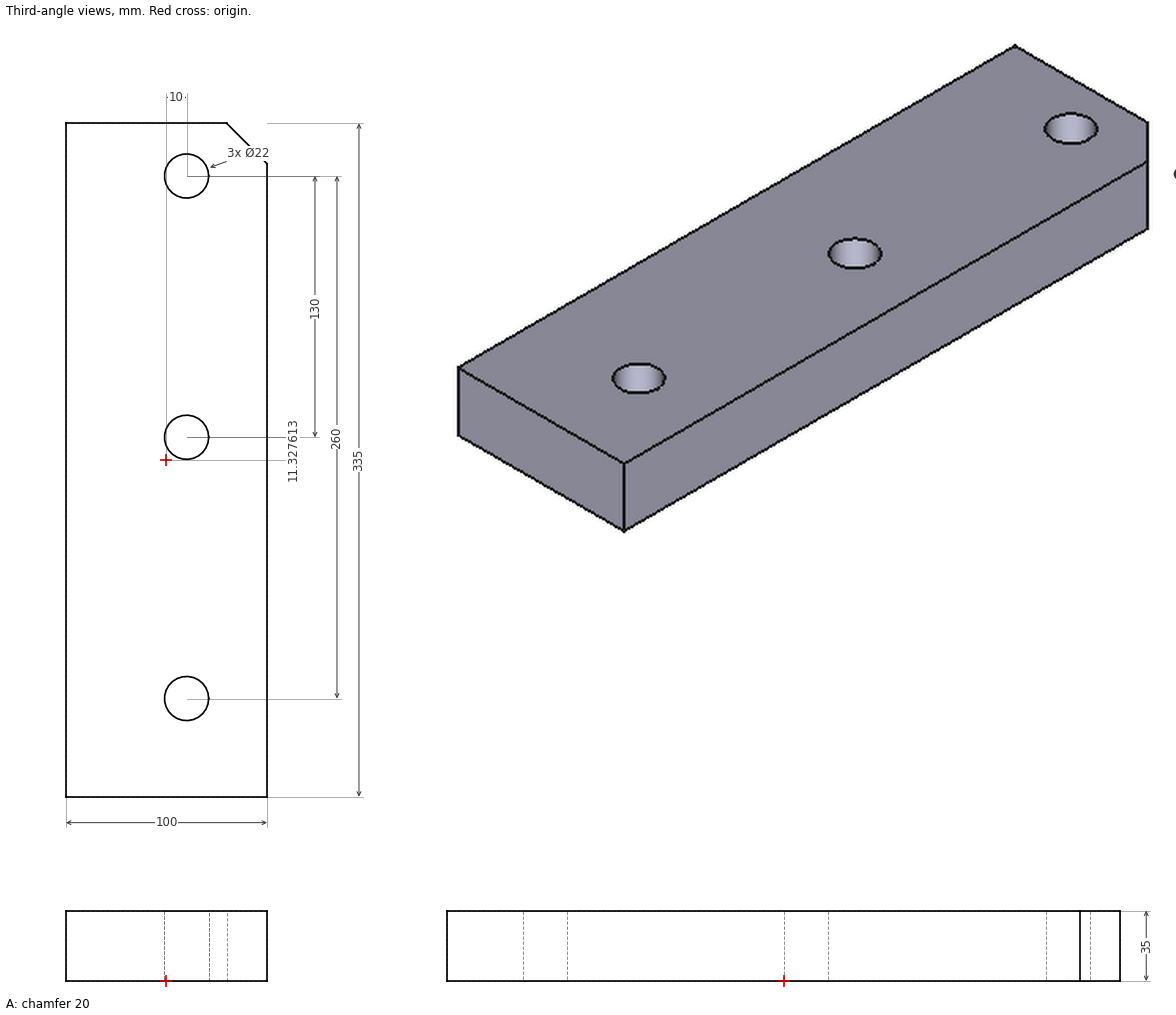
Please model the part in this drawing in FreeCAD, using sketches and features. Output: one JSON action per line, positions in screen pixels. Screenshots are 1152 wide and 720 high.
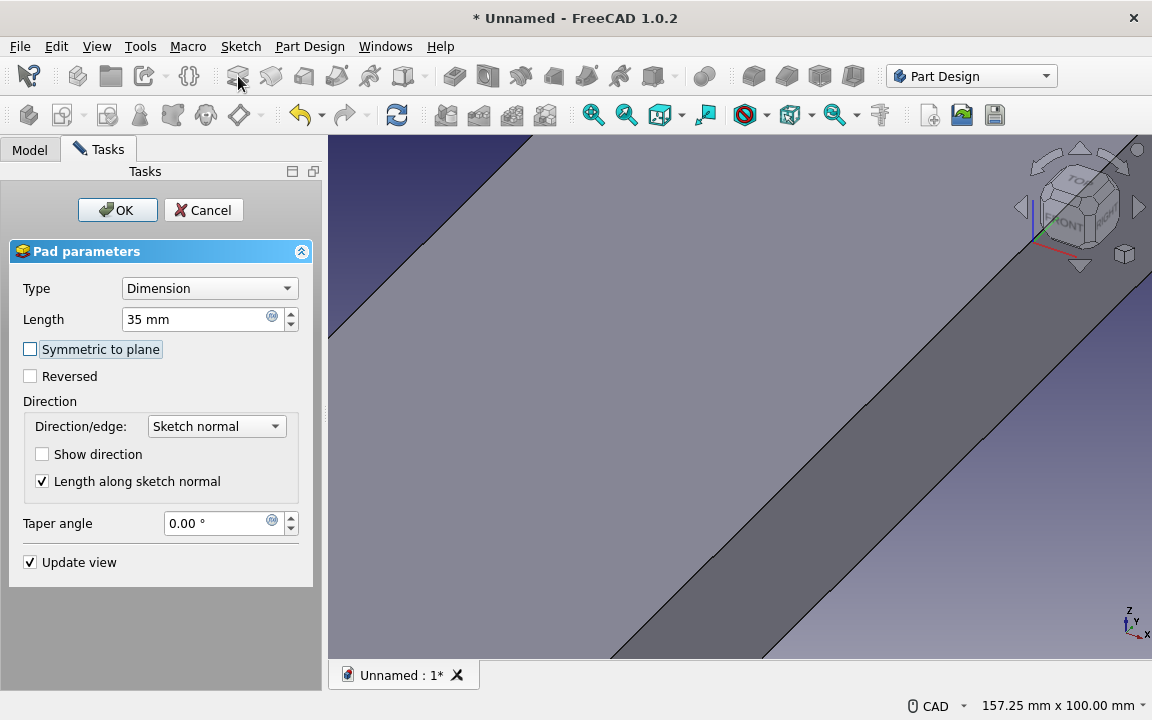
{"action": "left_click", "coordinate": [118, 210]}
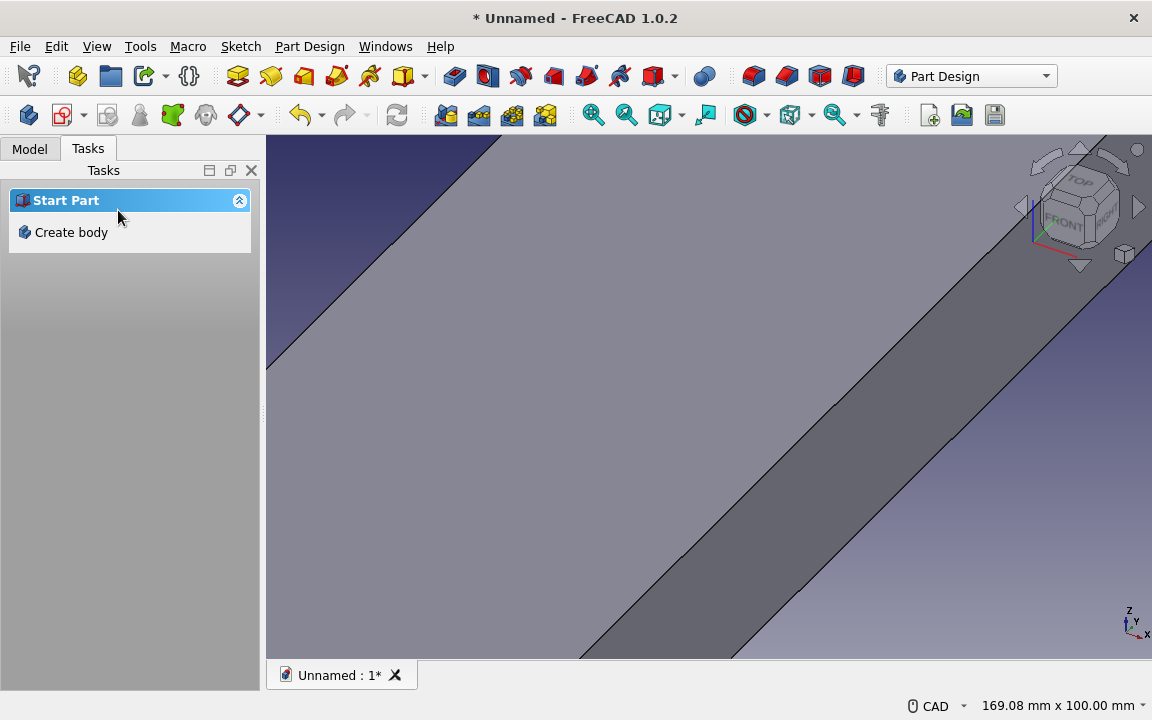
{"action": "left_click", "coordinate": [594, 116]}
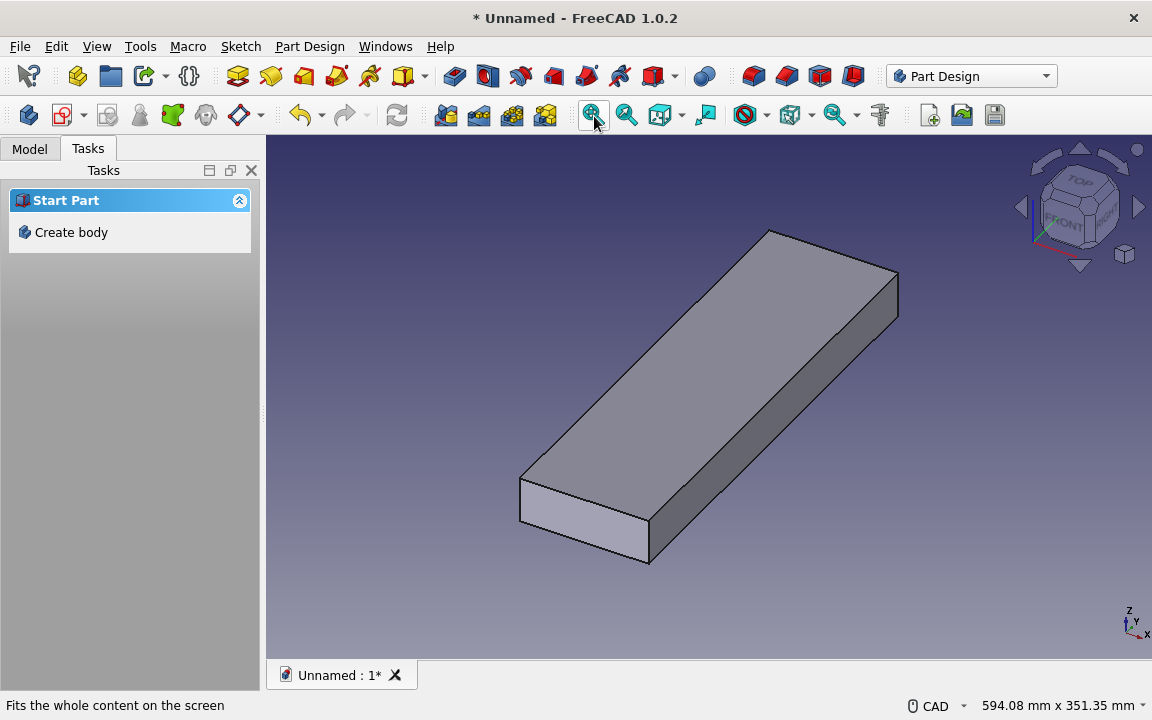
{"action": "key", "text": "0"}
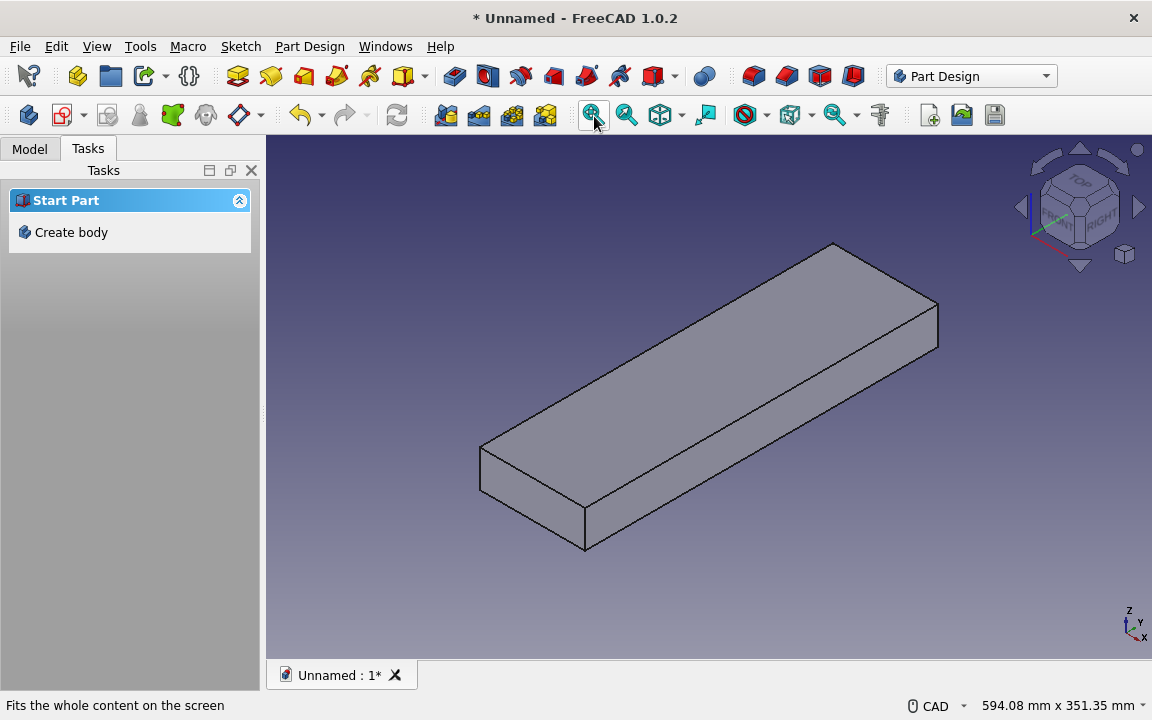
{"action": "key", "text": "2"}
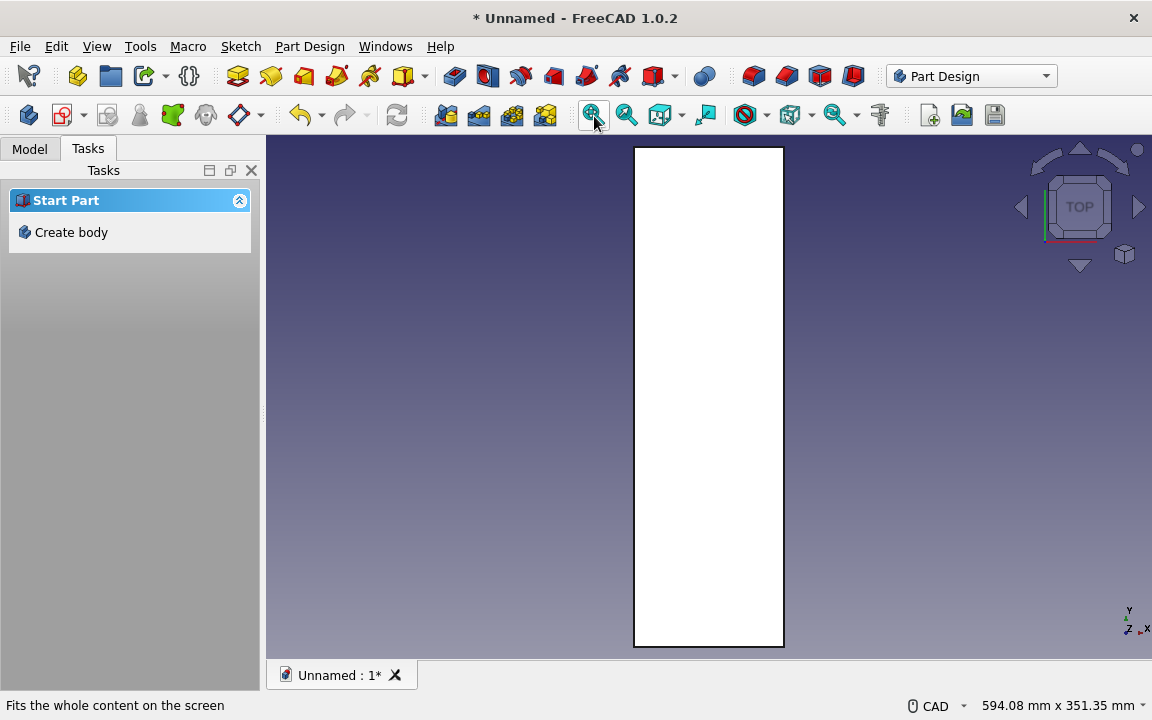
{"action": "key", "text": "1"}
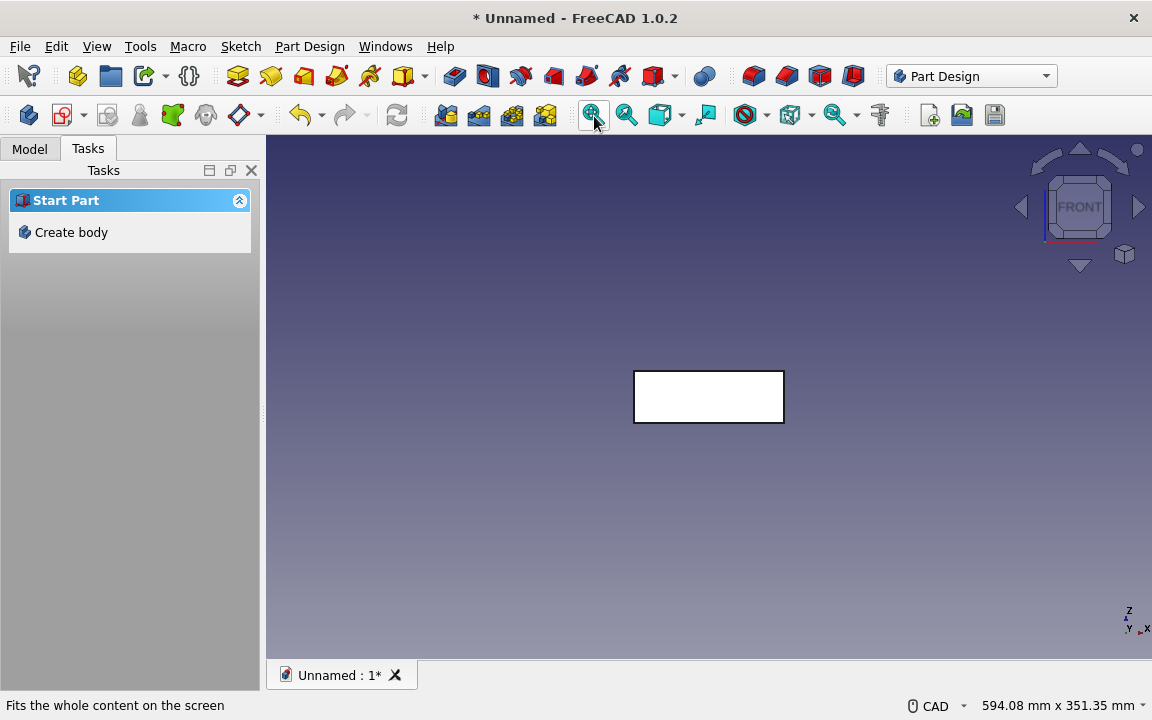
{"action": "left_click", "coordinate": [594, 116]}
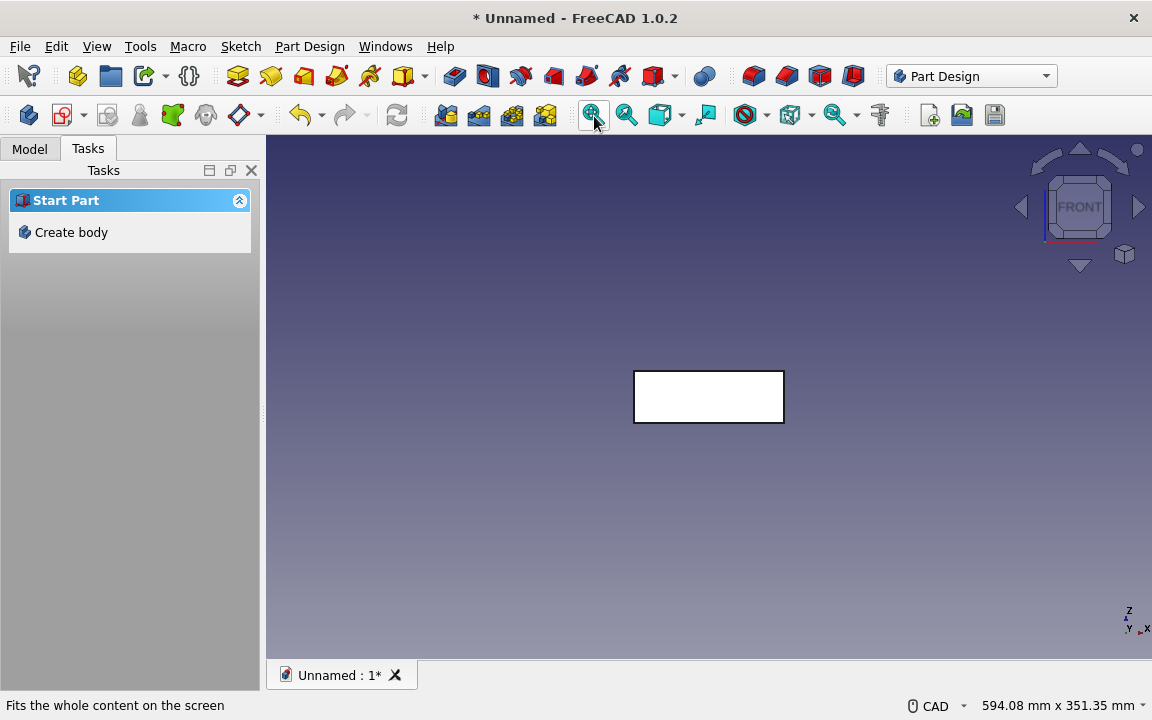
{"action": "key", "text": "3"}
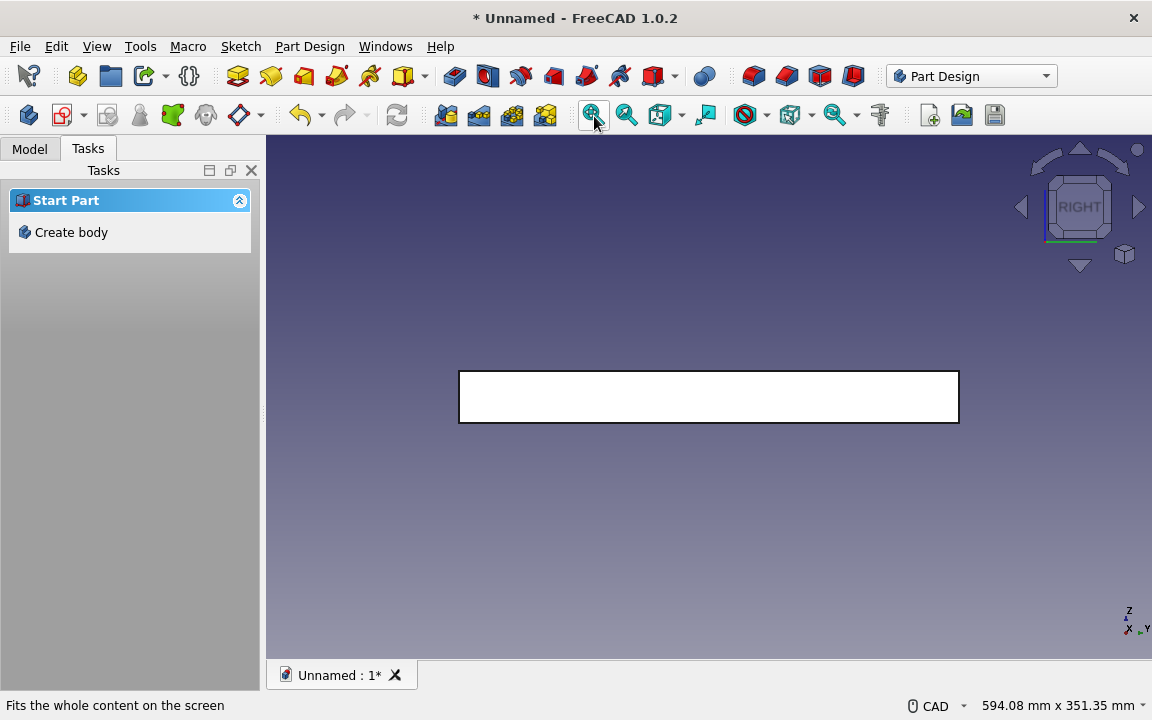
{"action": "left_click", "coordinate": [959, 396]}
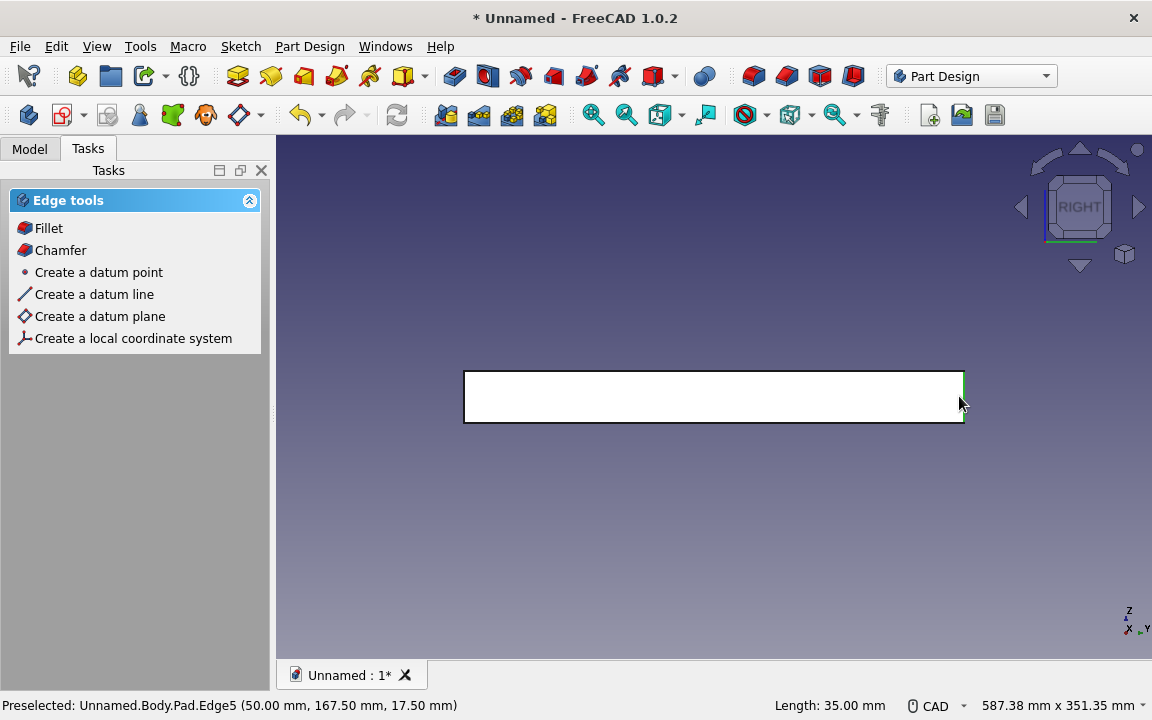
{"action": "left_click", "coordinate": [787, 76]}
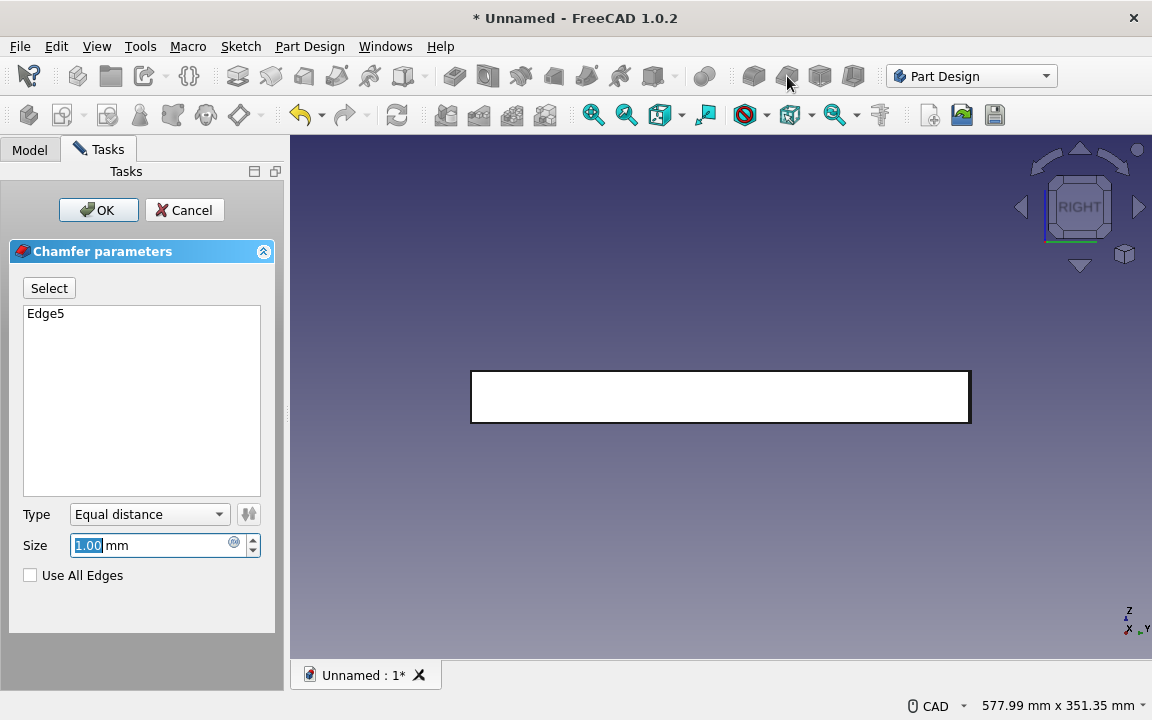
{"action": "type", "text": "20"}
{"action": "key", "text": "Tab"}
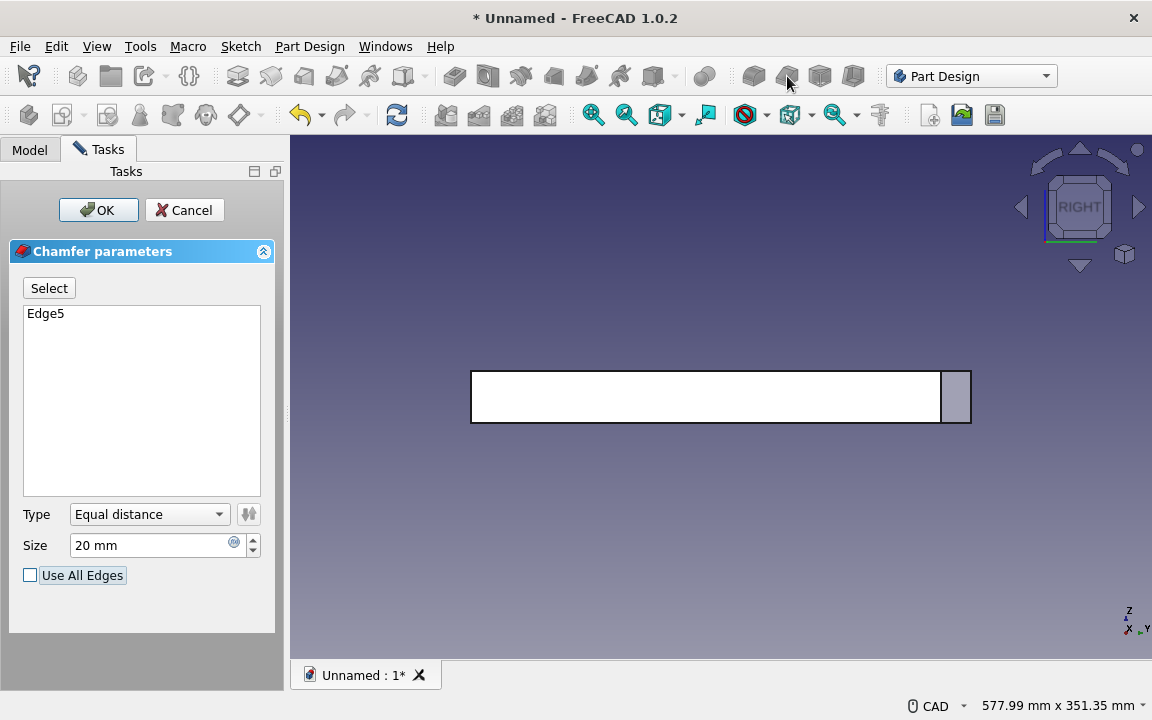
{"action": "left_click", "coordinate": [99, 210]}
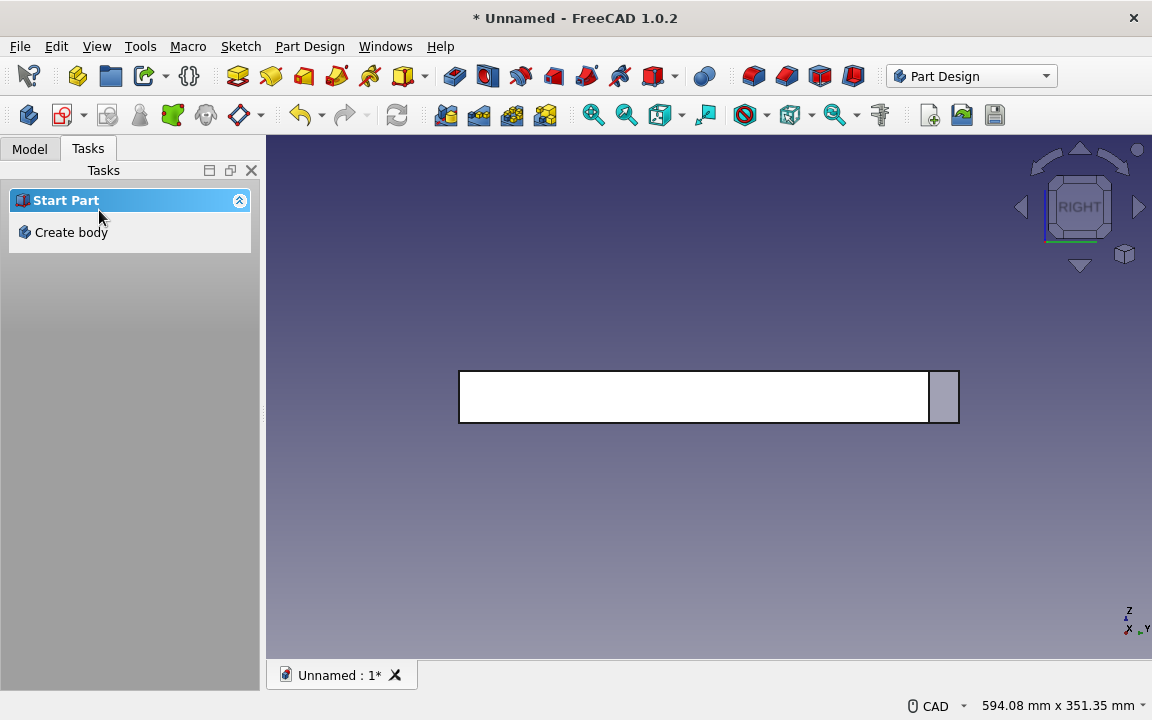
{"action": "key", "text": "0"}